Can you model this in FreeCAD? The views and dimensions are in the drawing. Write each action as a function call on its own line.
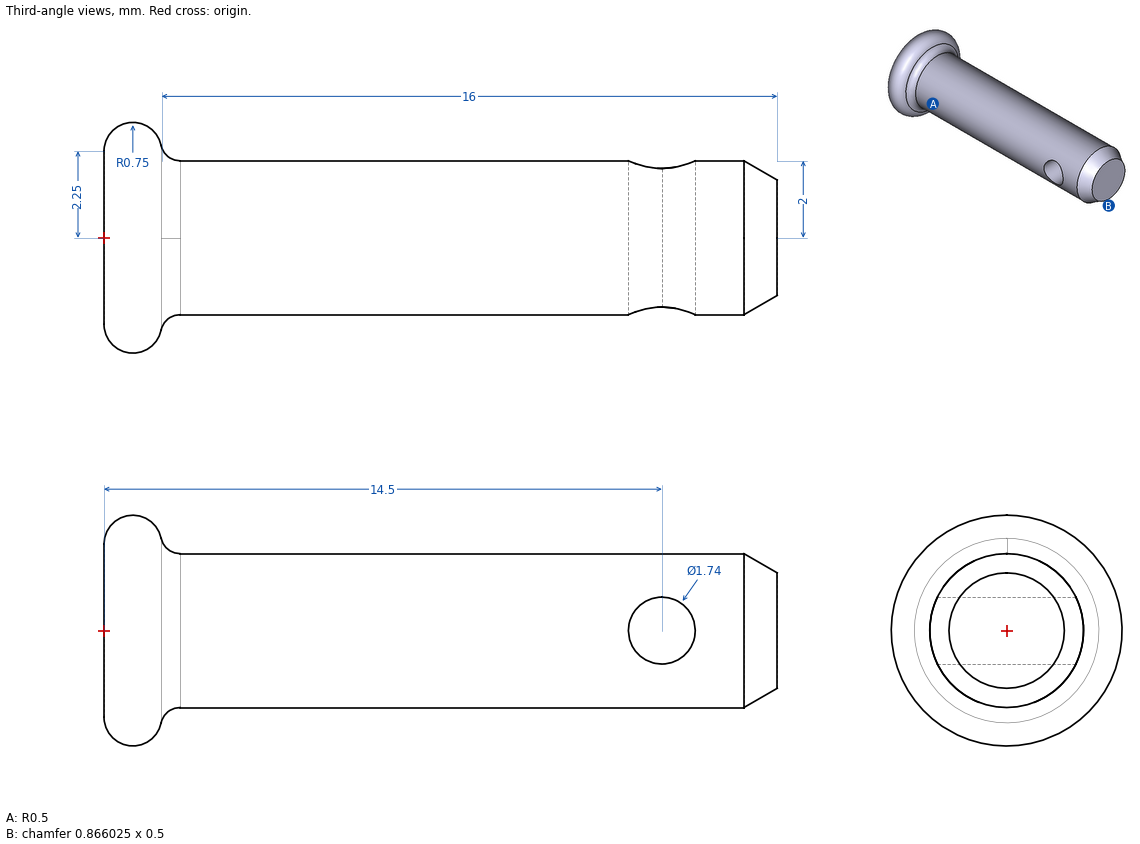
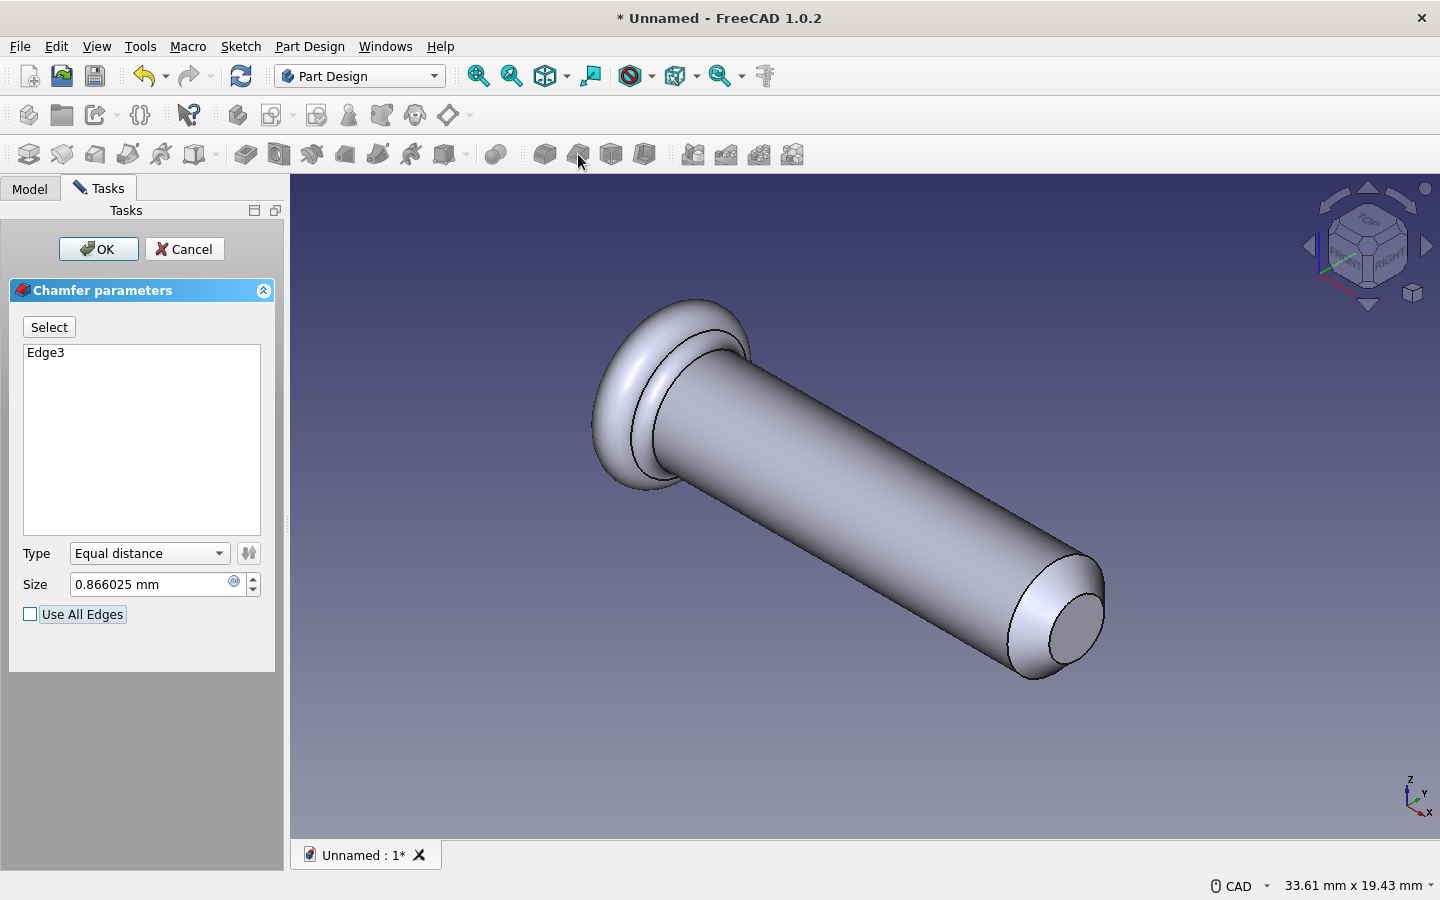
click(150, 554)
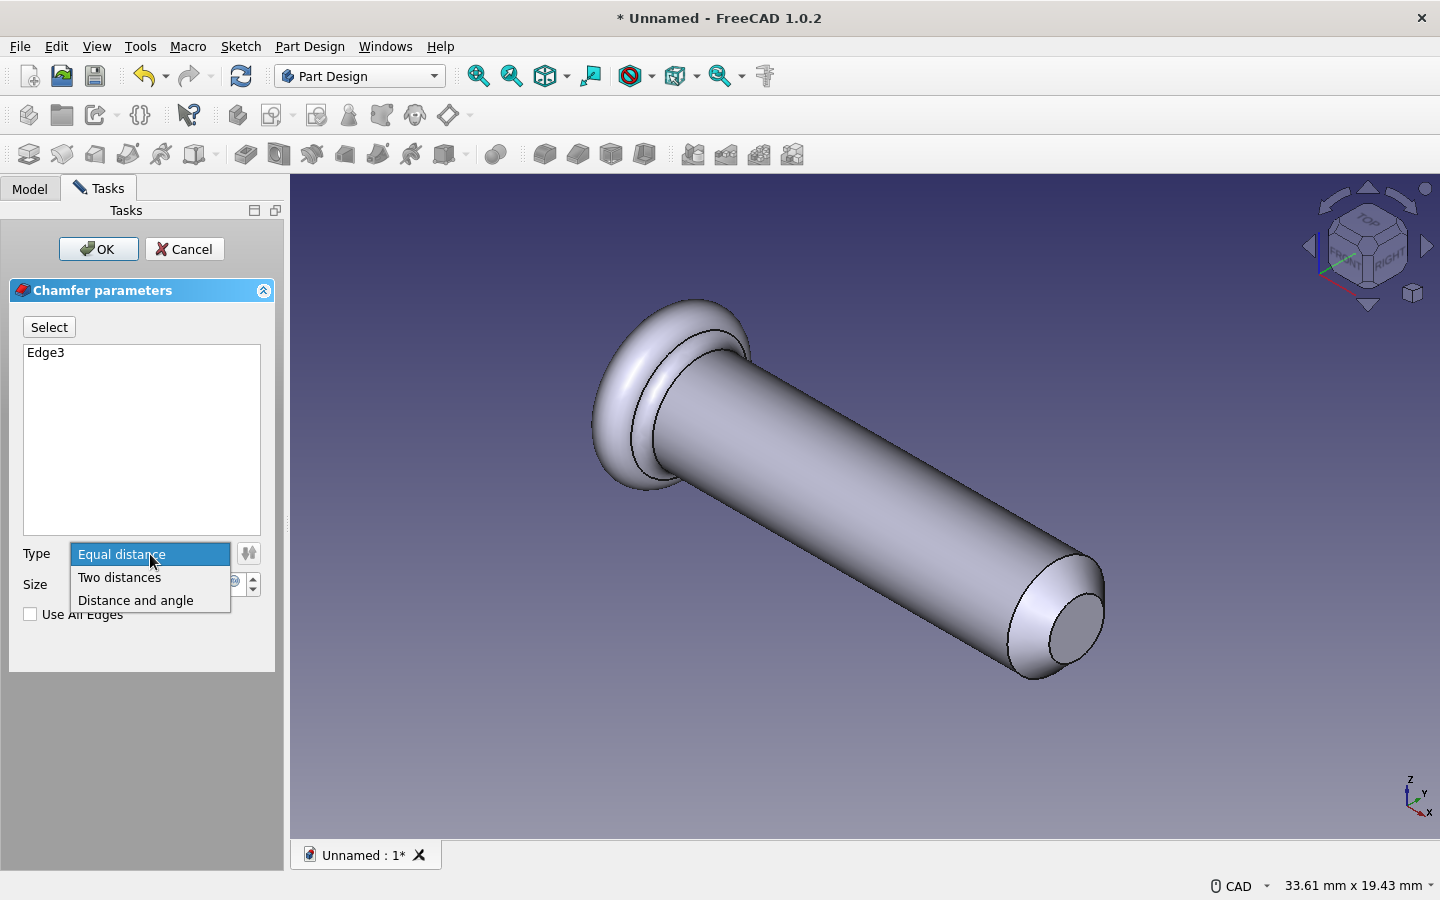
click(148, 578)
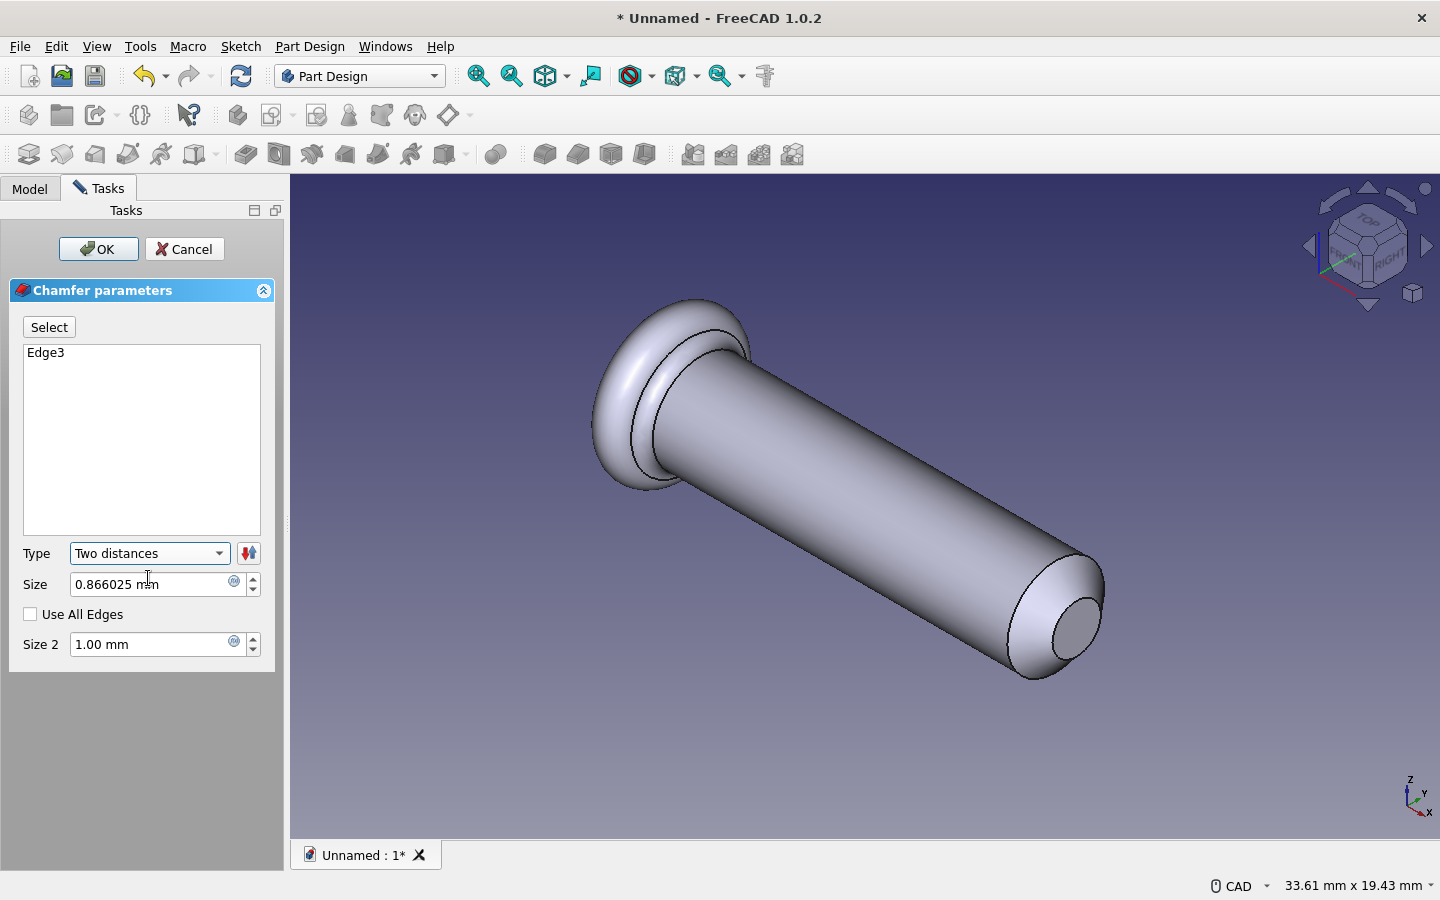
triple_click(158, 644)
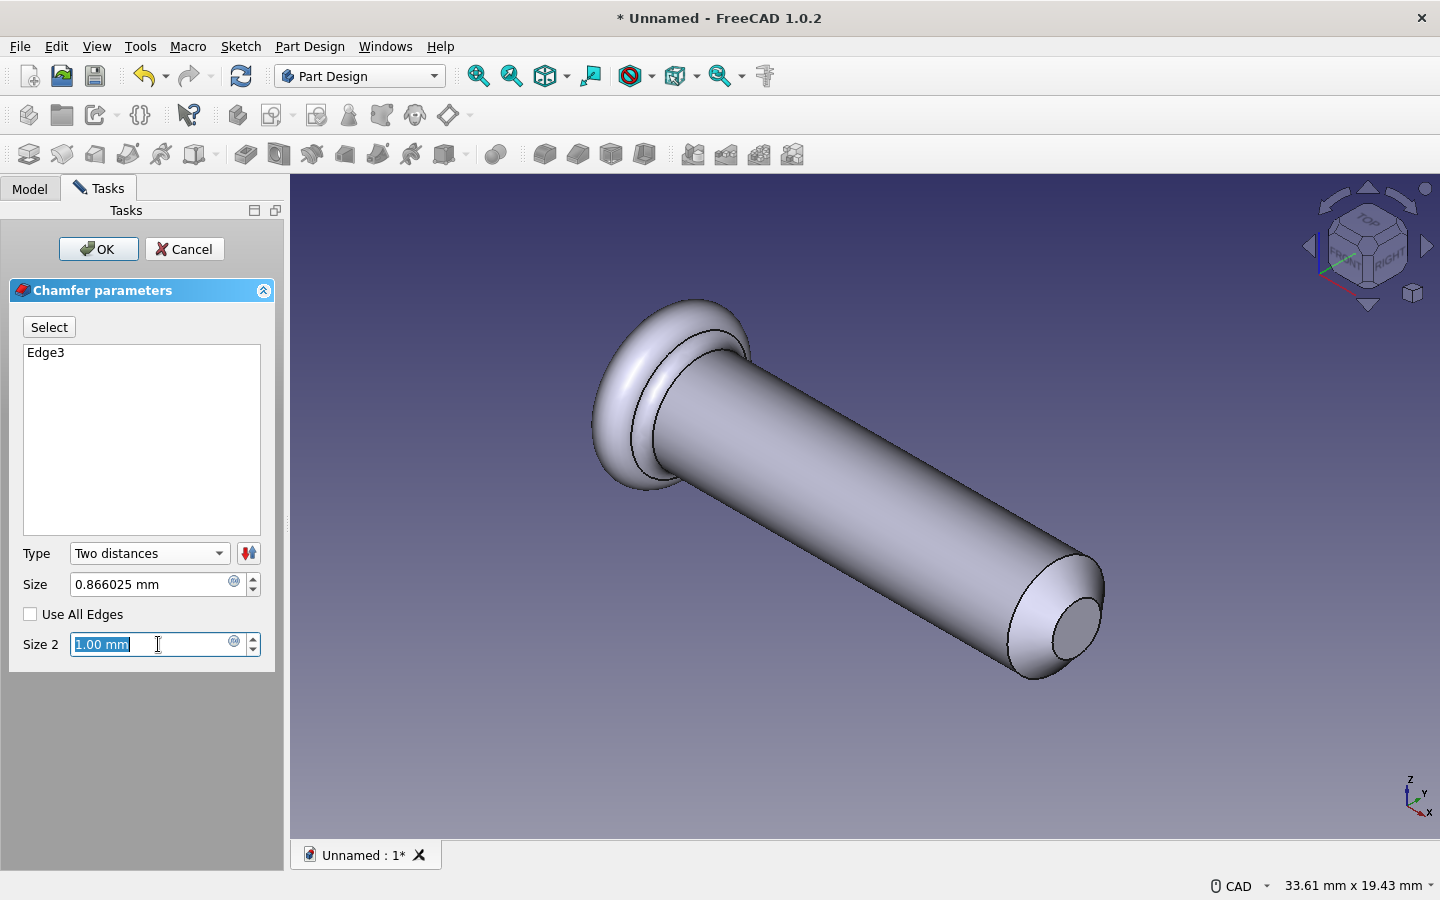
text(0.5)
key(Tab)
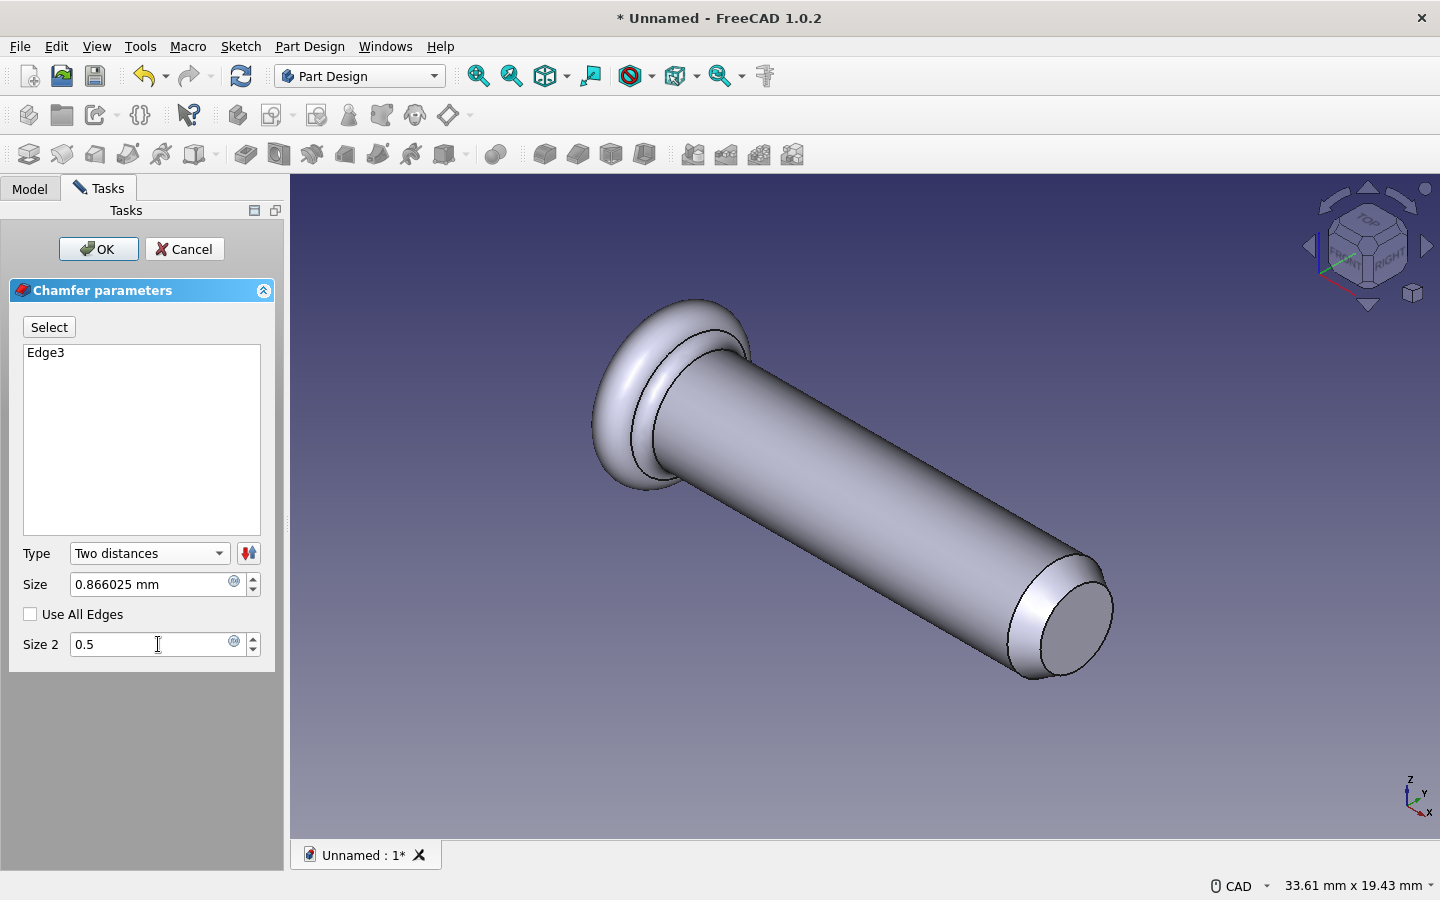
click(99, 249)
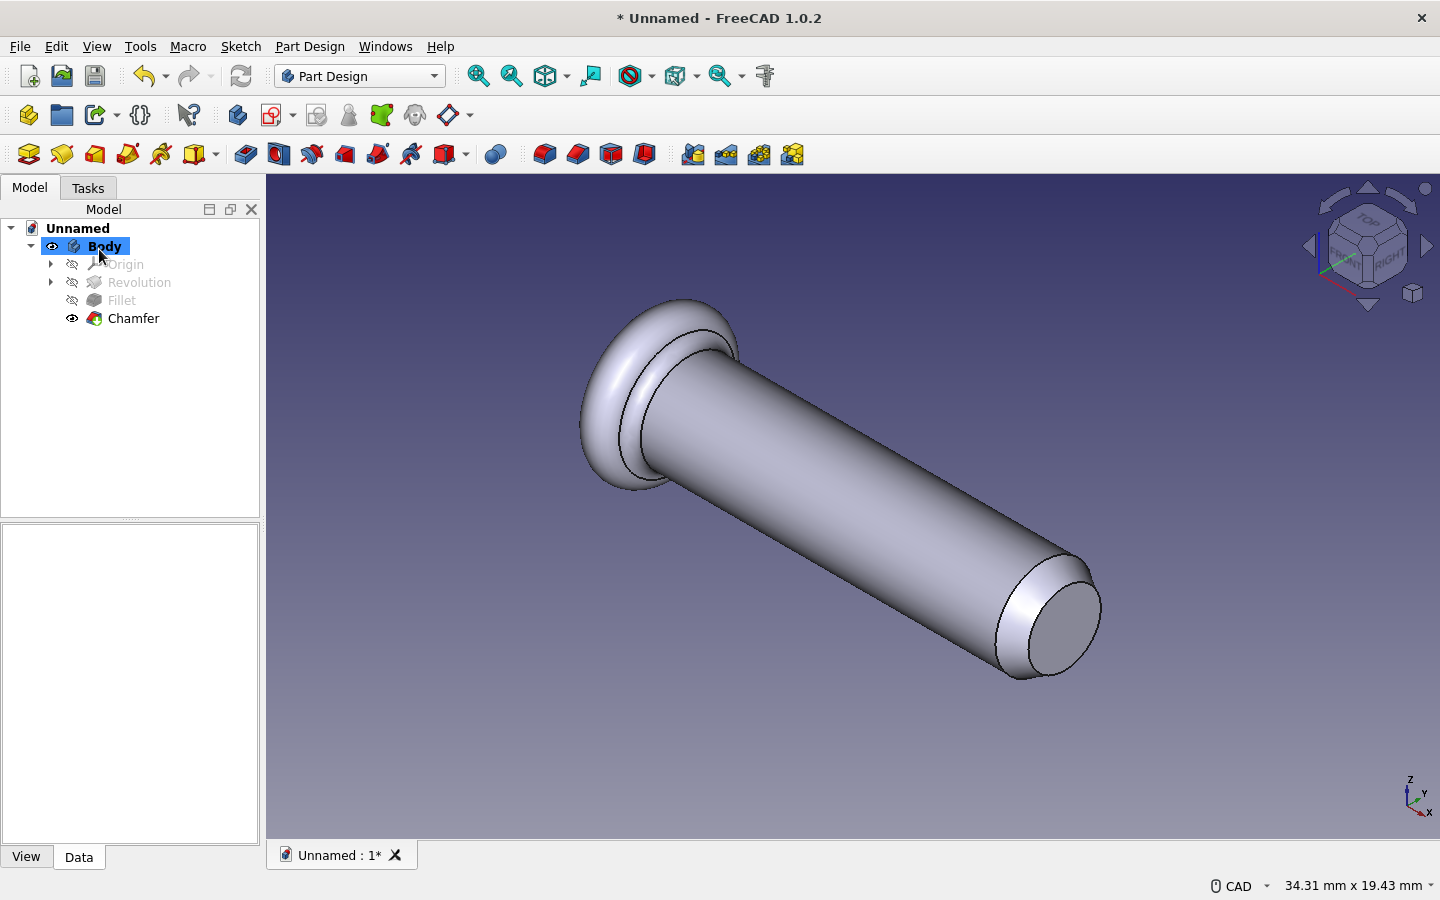
click(270, 116)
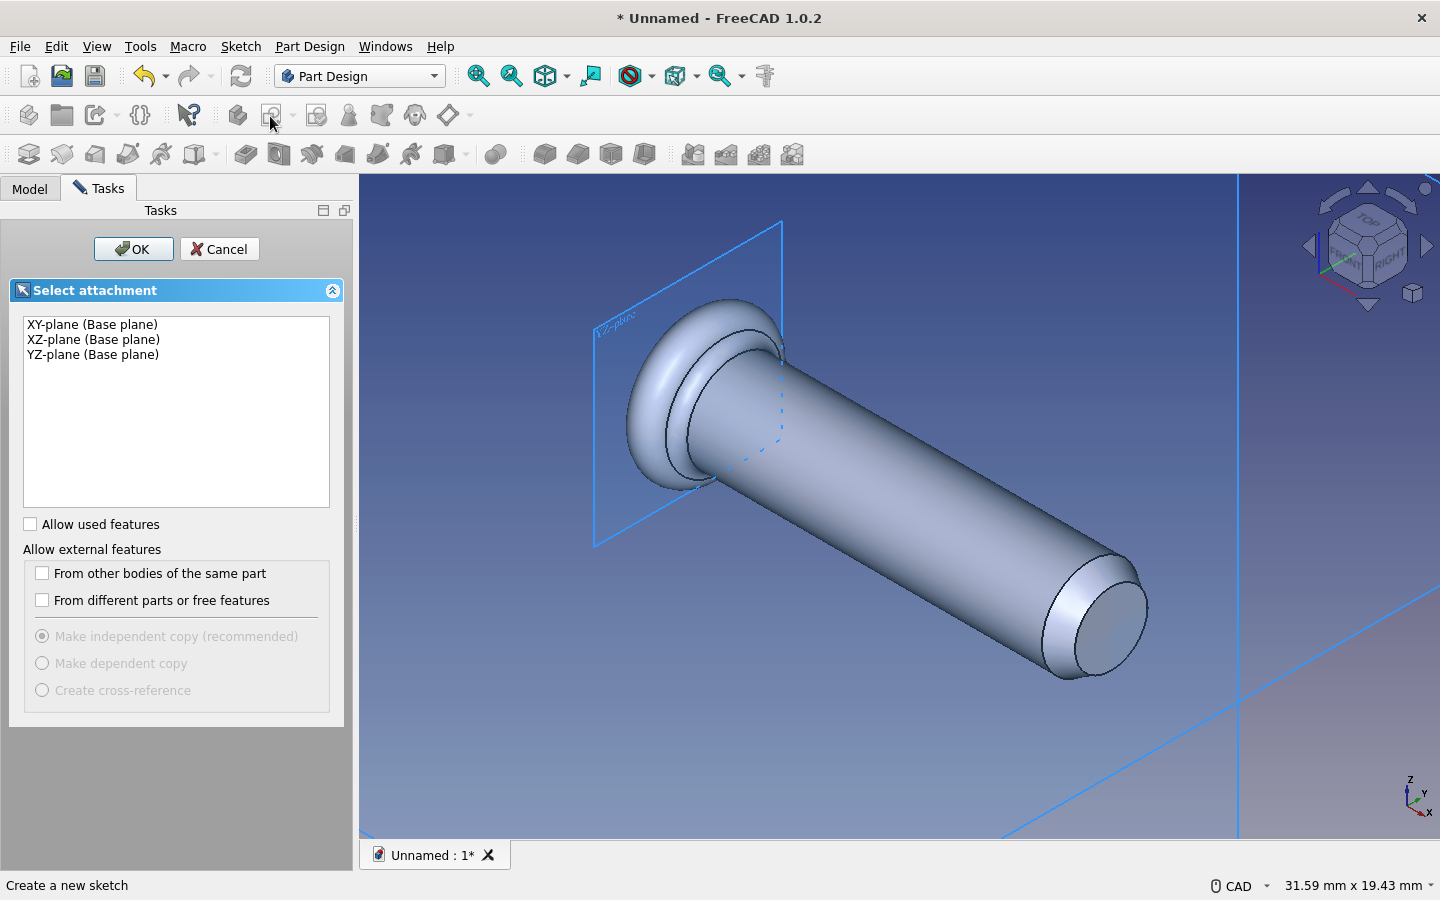
click(84, 340)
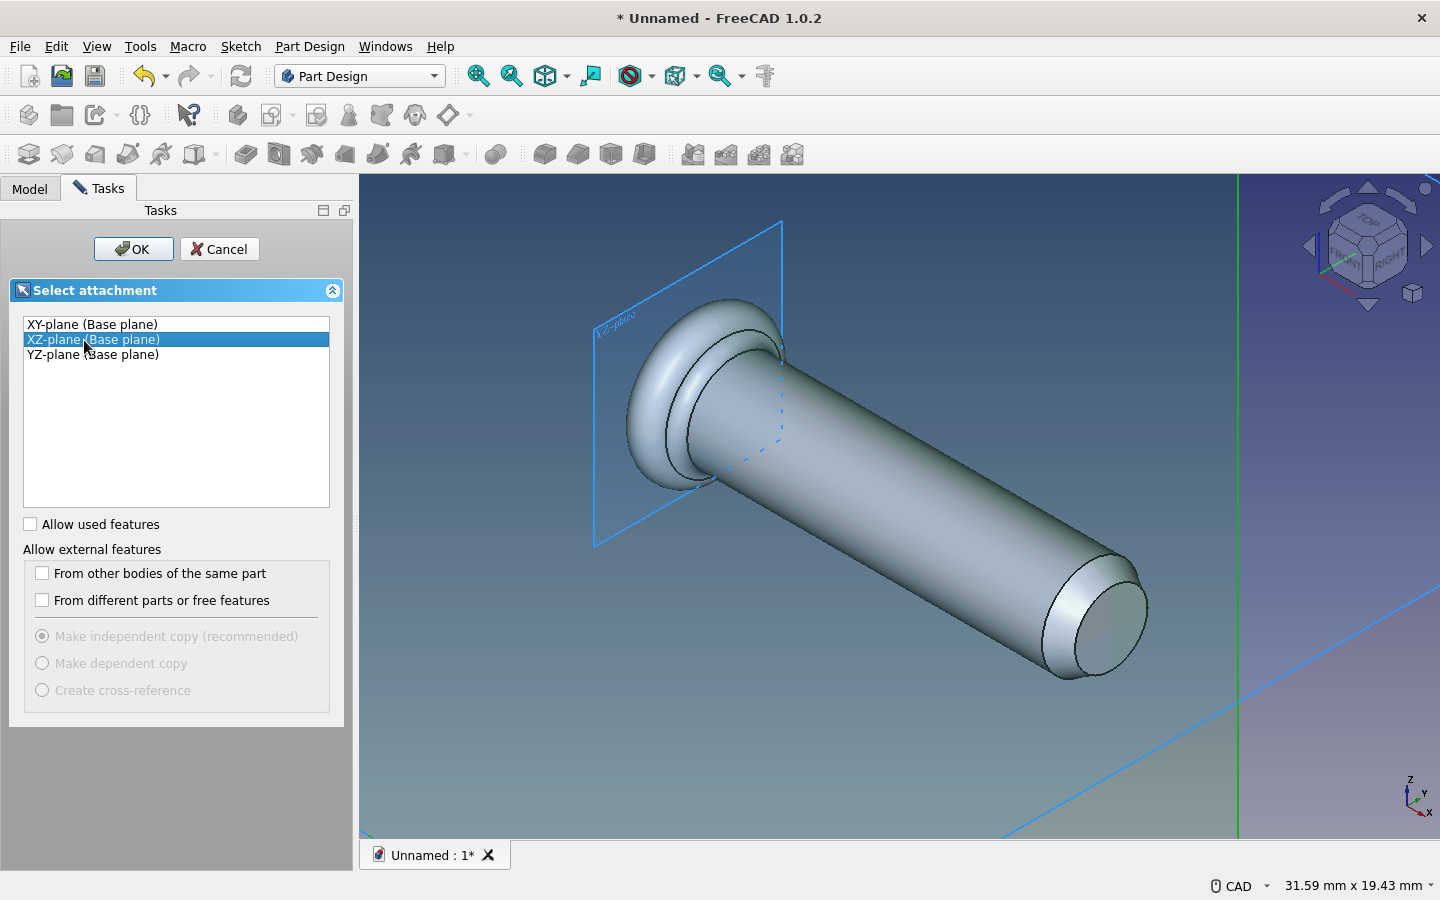
click(134, 249)